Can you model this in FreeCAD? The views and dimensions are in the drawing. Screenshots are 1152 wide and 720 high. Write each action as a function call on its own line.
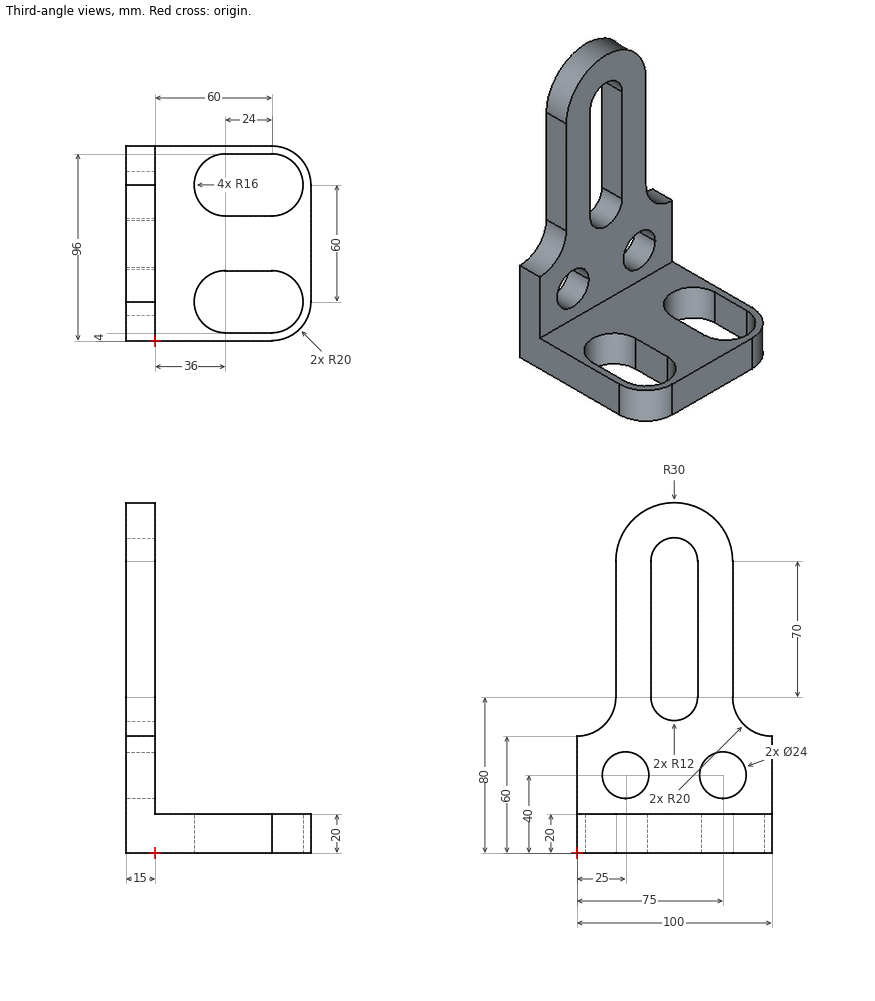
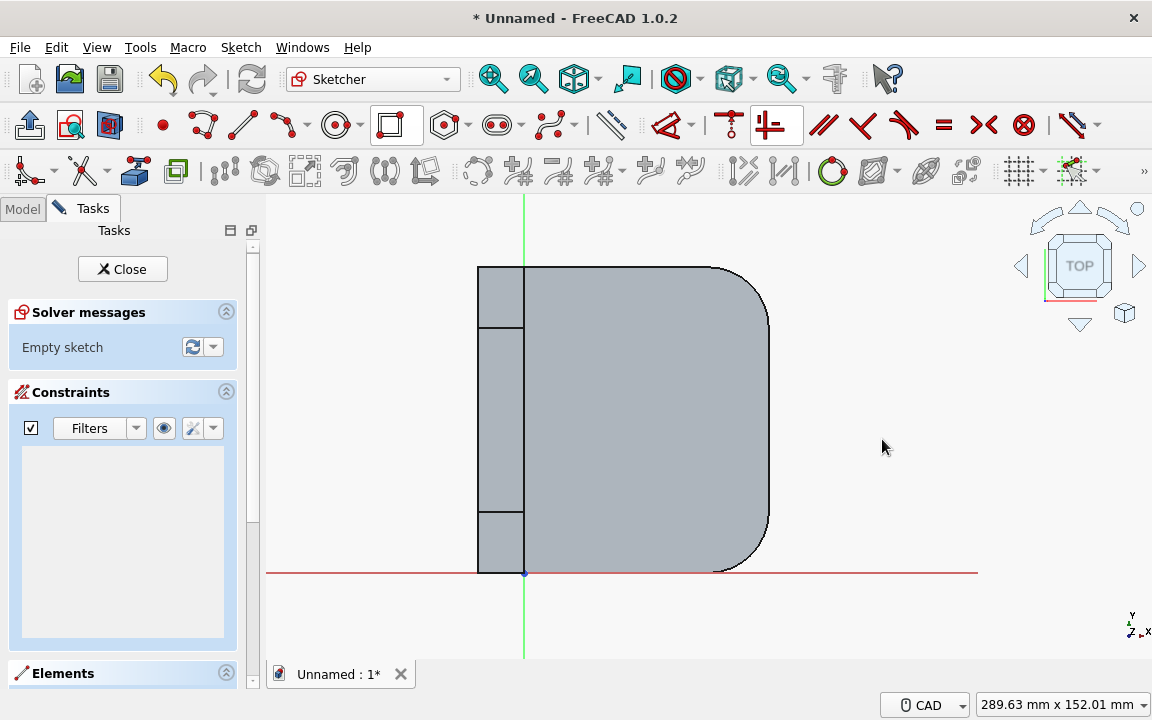
click(634, 328)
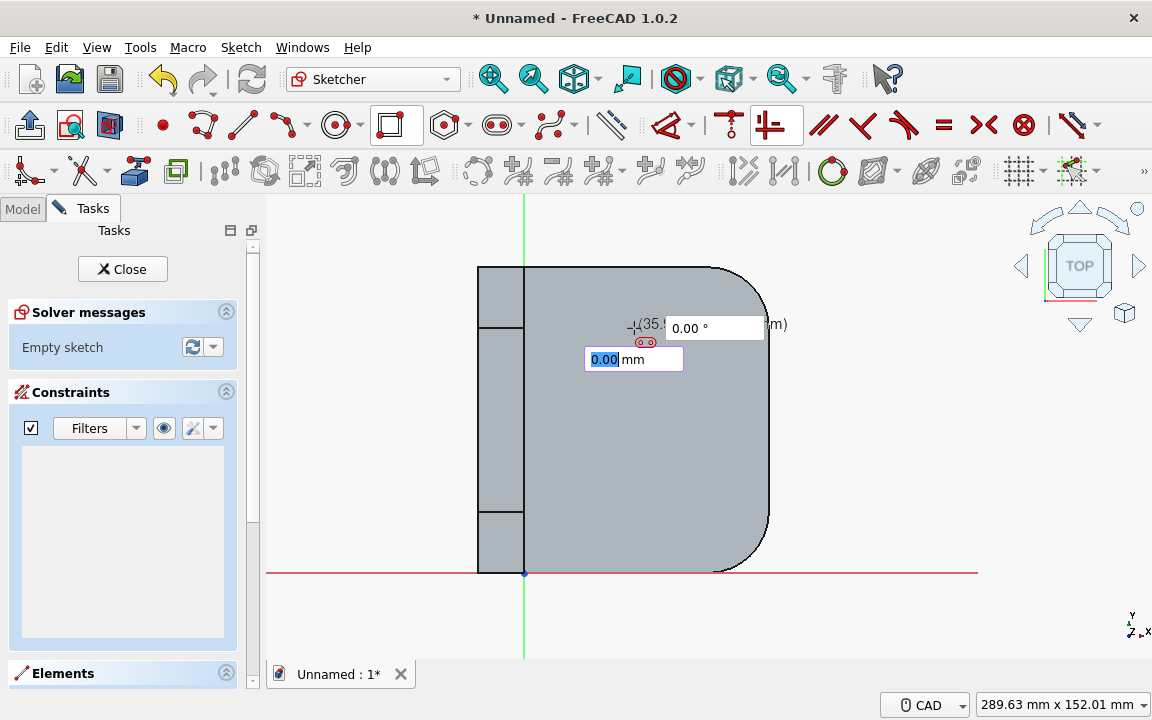
click(708, 328)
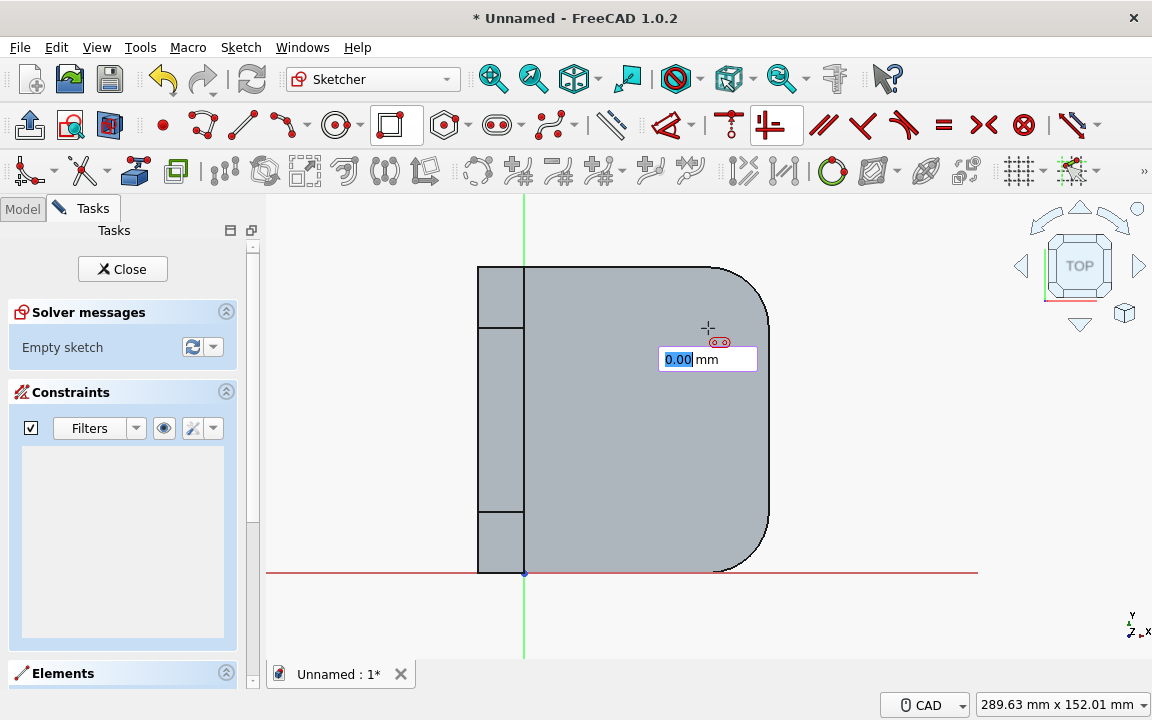
click(671, 279)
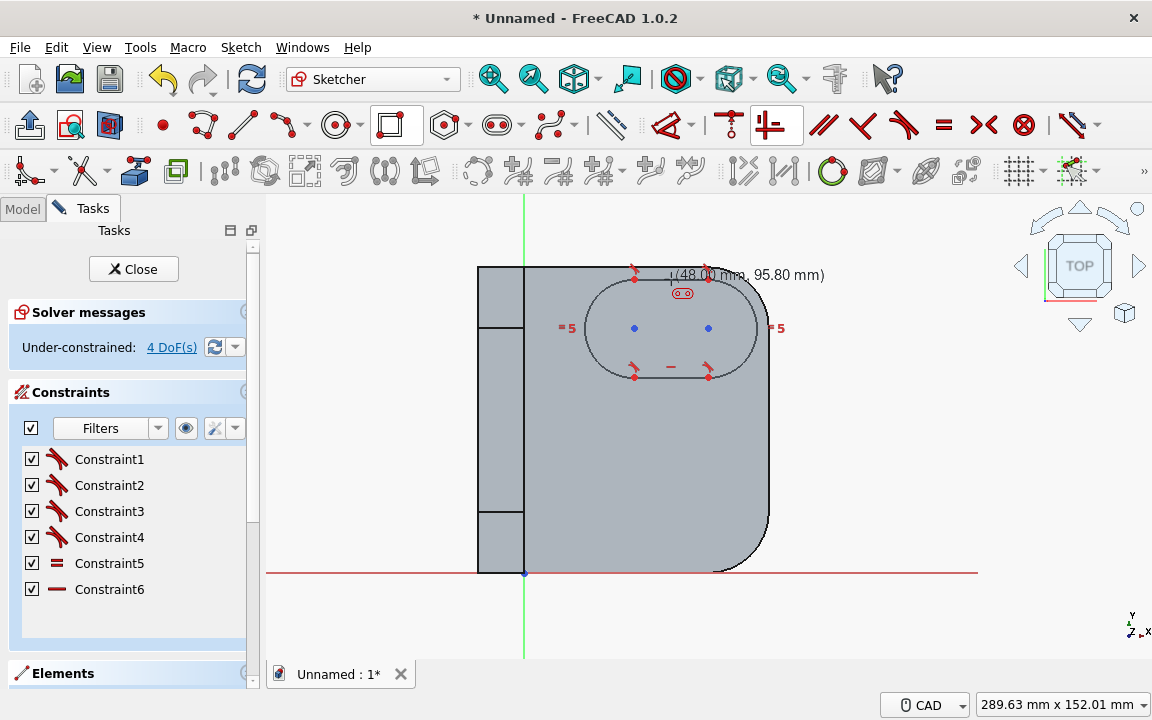
click(634, 512)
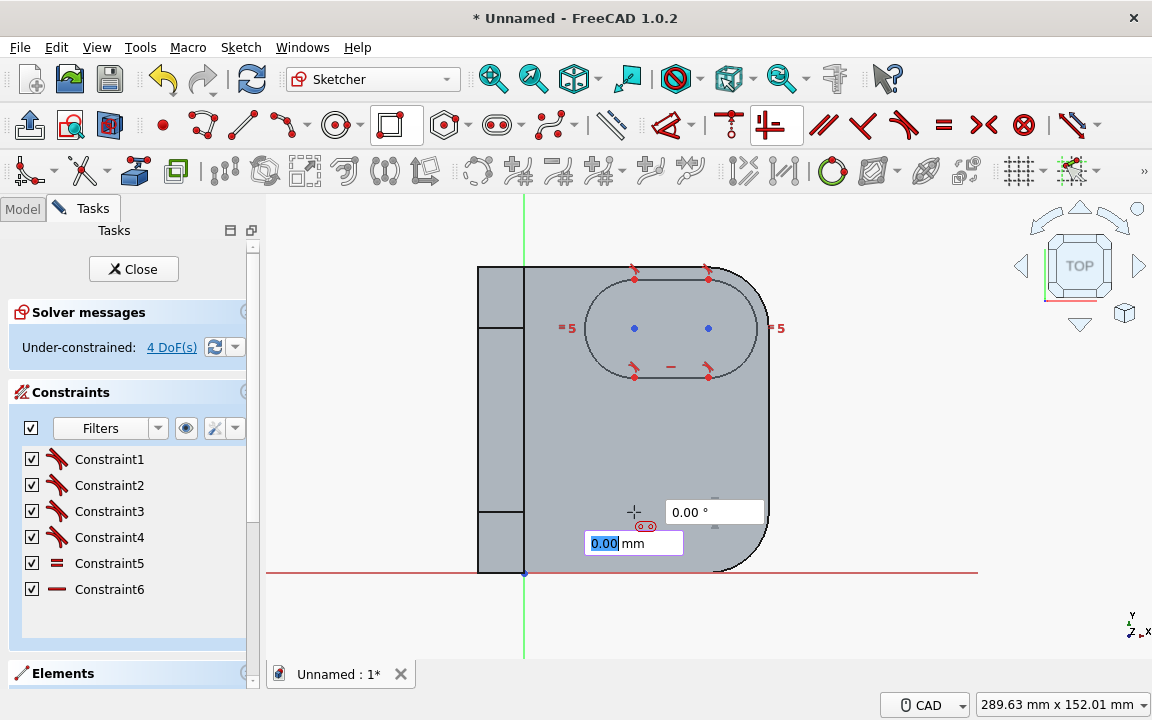
click(708, 512)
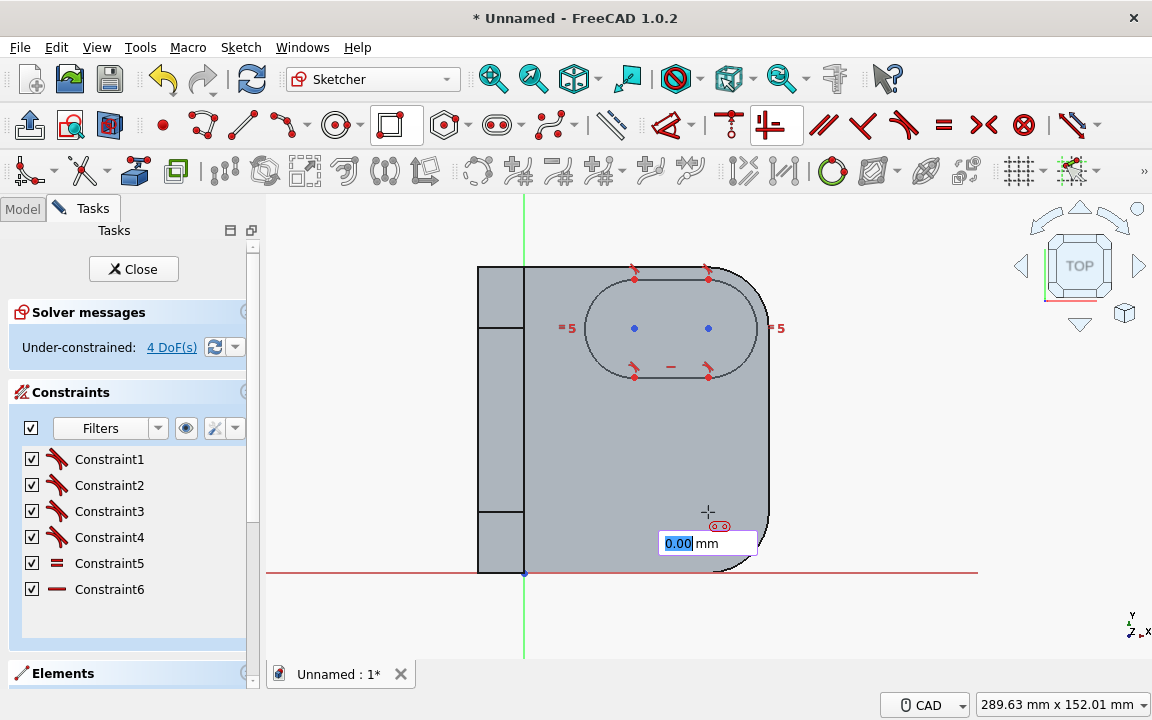
click(671, 463)
key(Escape)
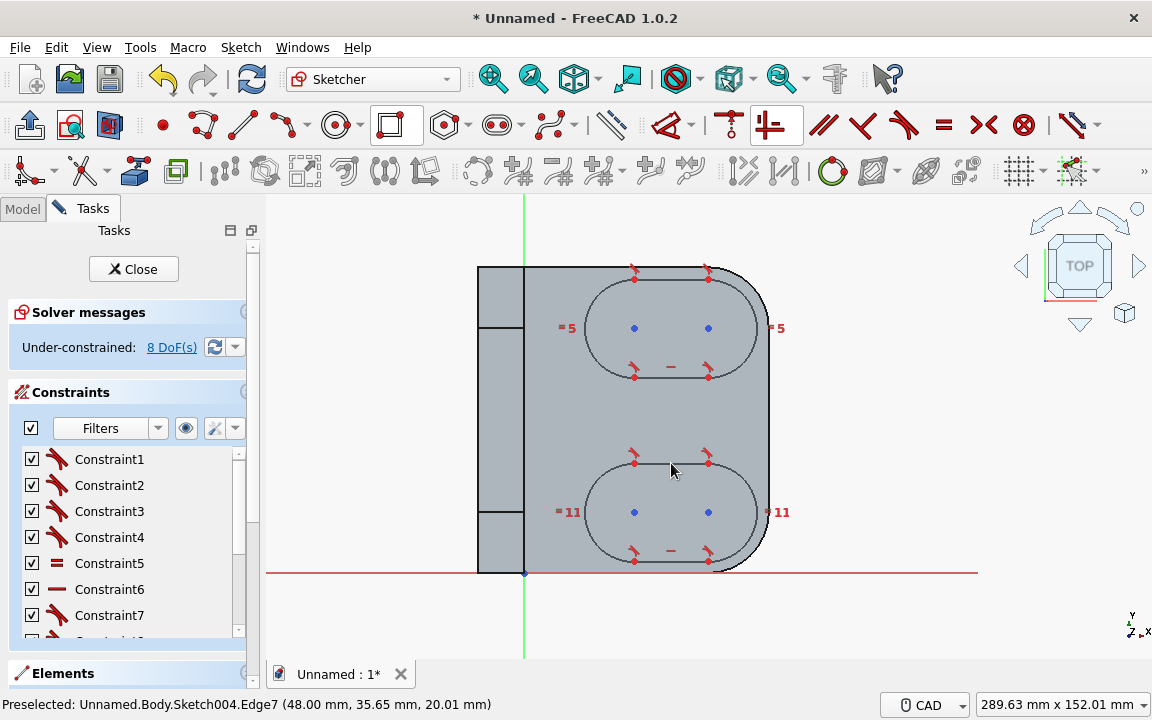
click(594, 300)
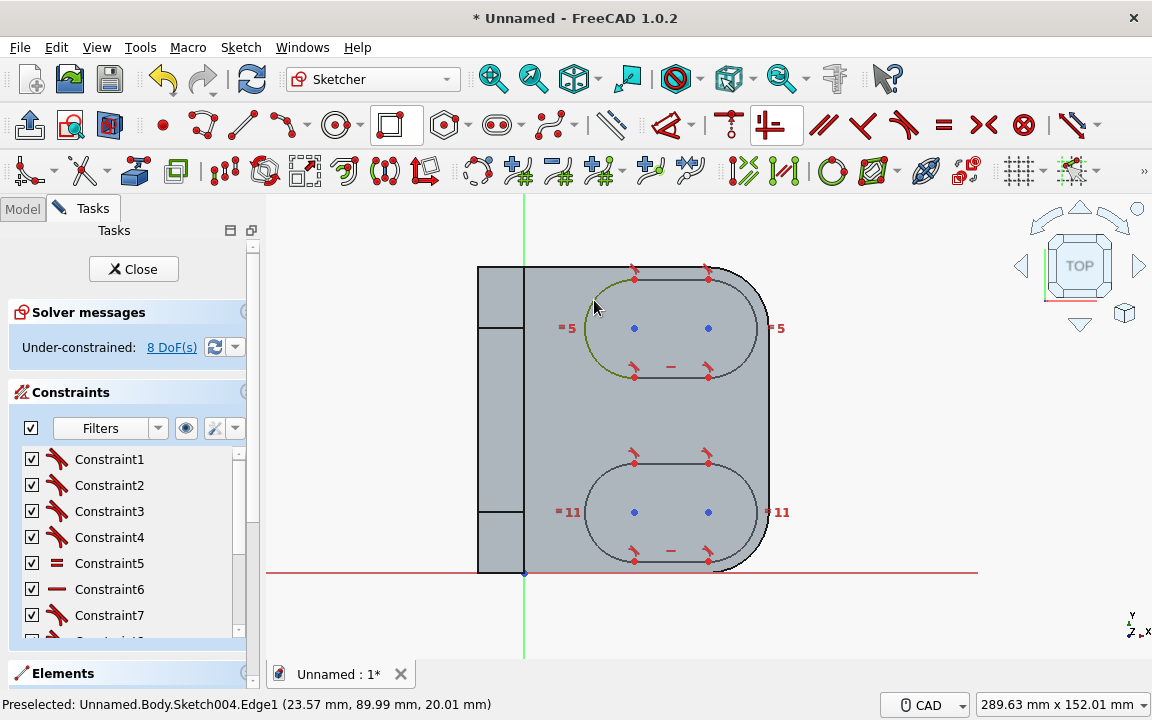
click(594, 484)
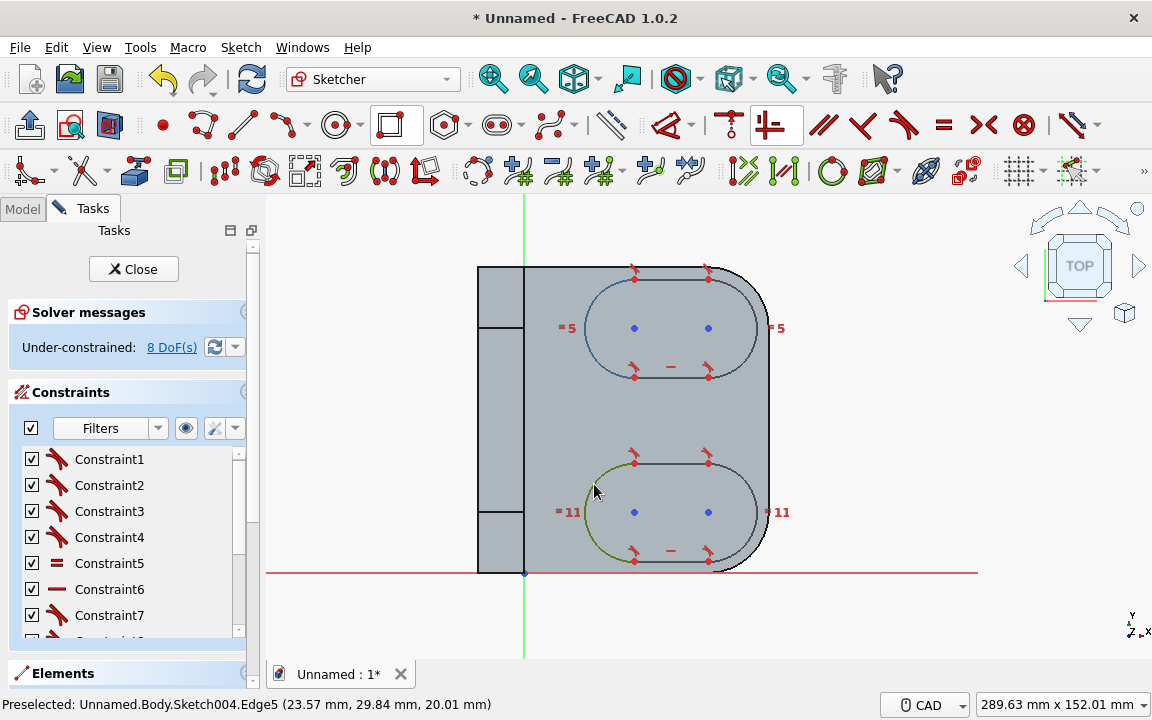
click(944, 126)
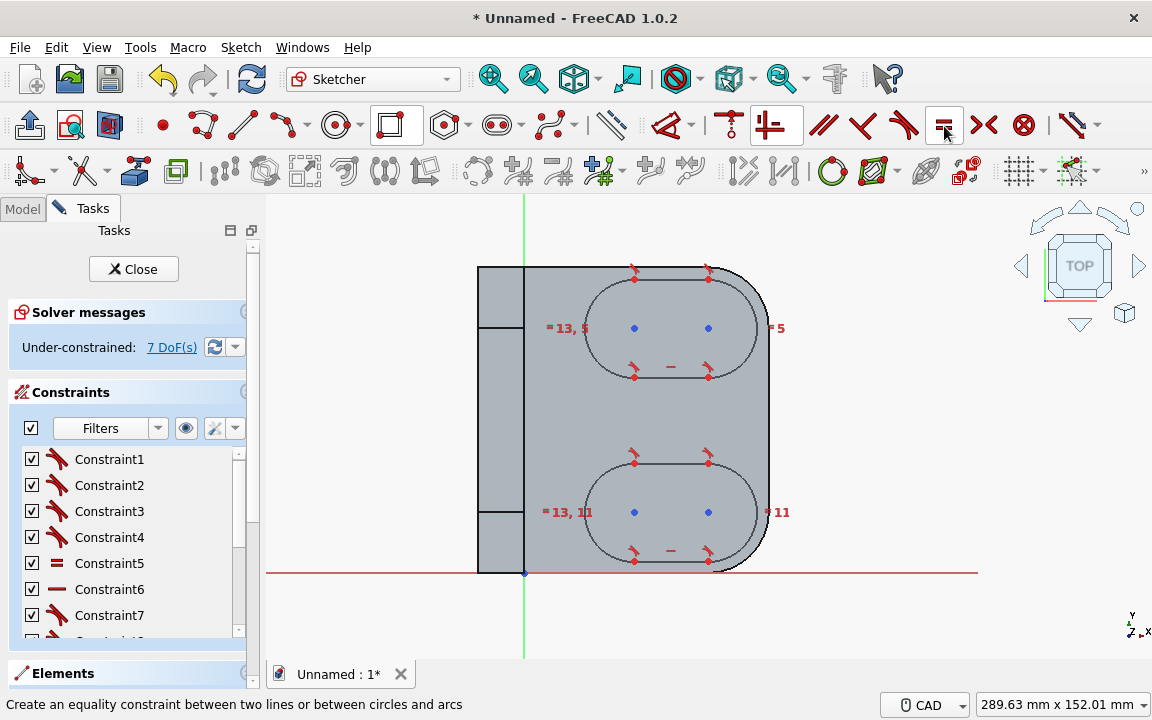
key(d)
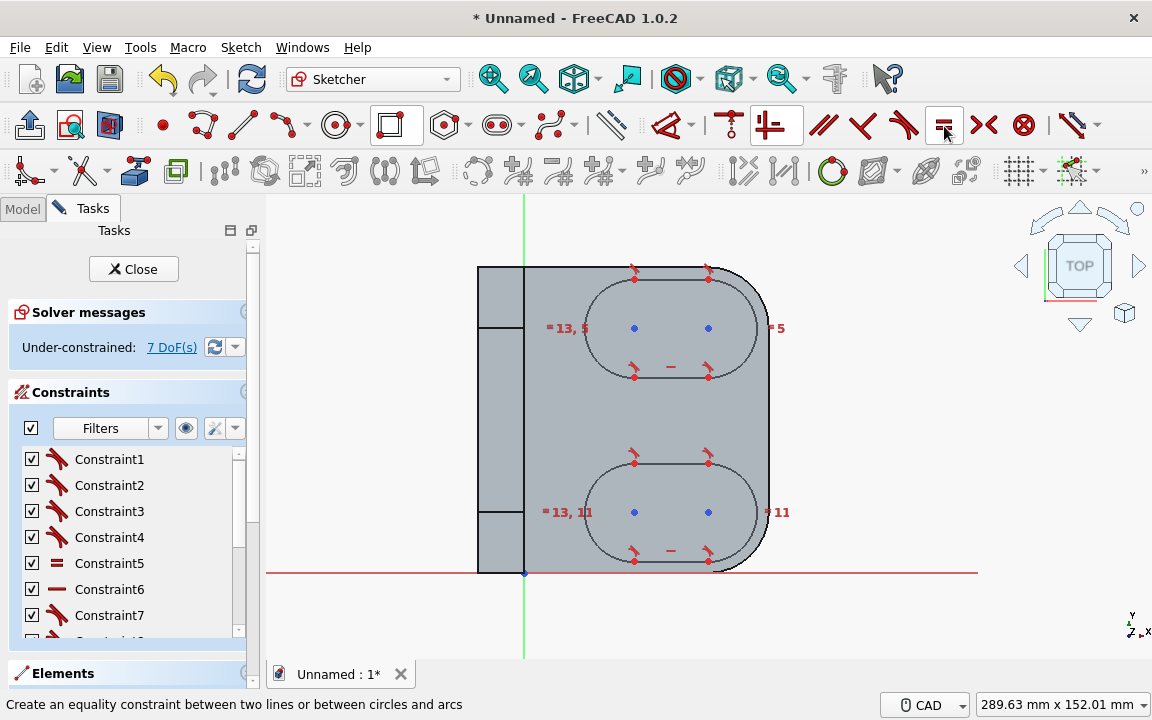
click(594, 300)
click(568, 281)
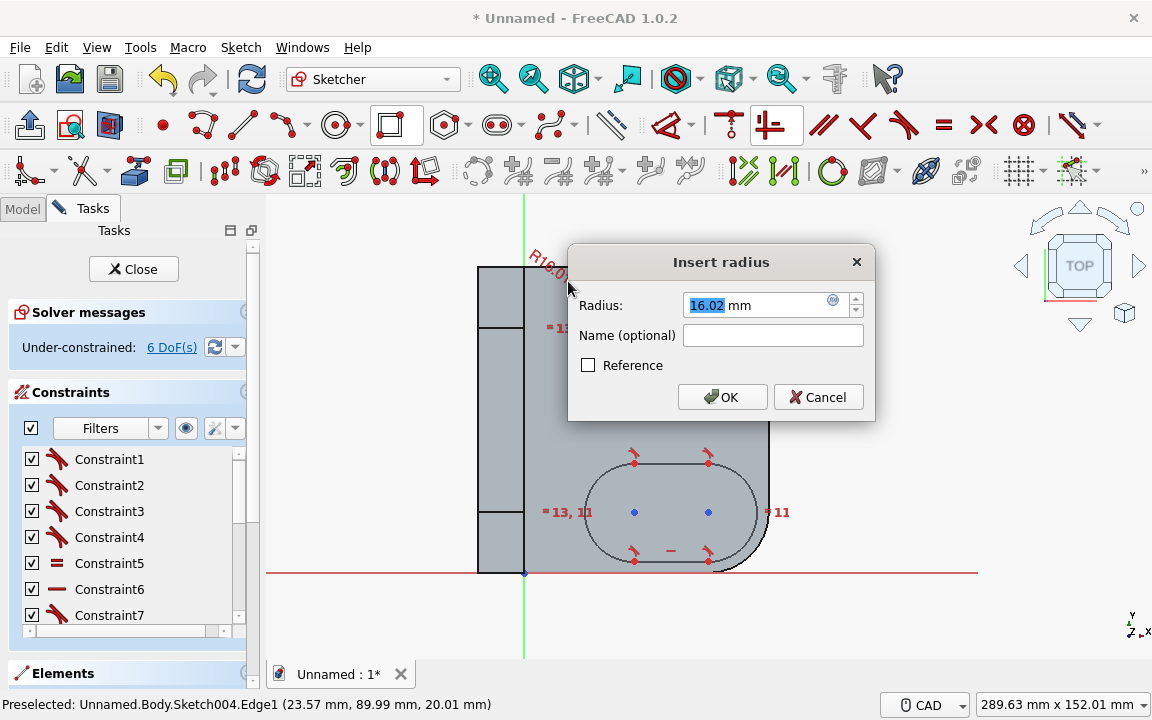
text(16)
key(Return)